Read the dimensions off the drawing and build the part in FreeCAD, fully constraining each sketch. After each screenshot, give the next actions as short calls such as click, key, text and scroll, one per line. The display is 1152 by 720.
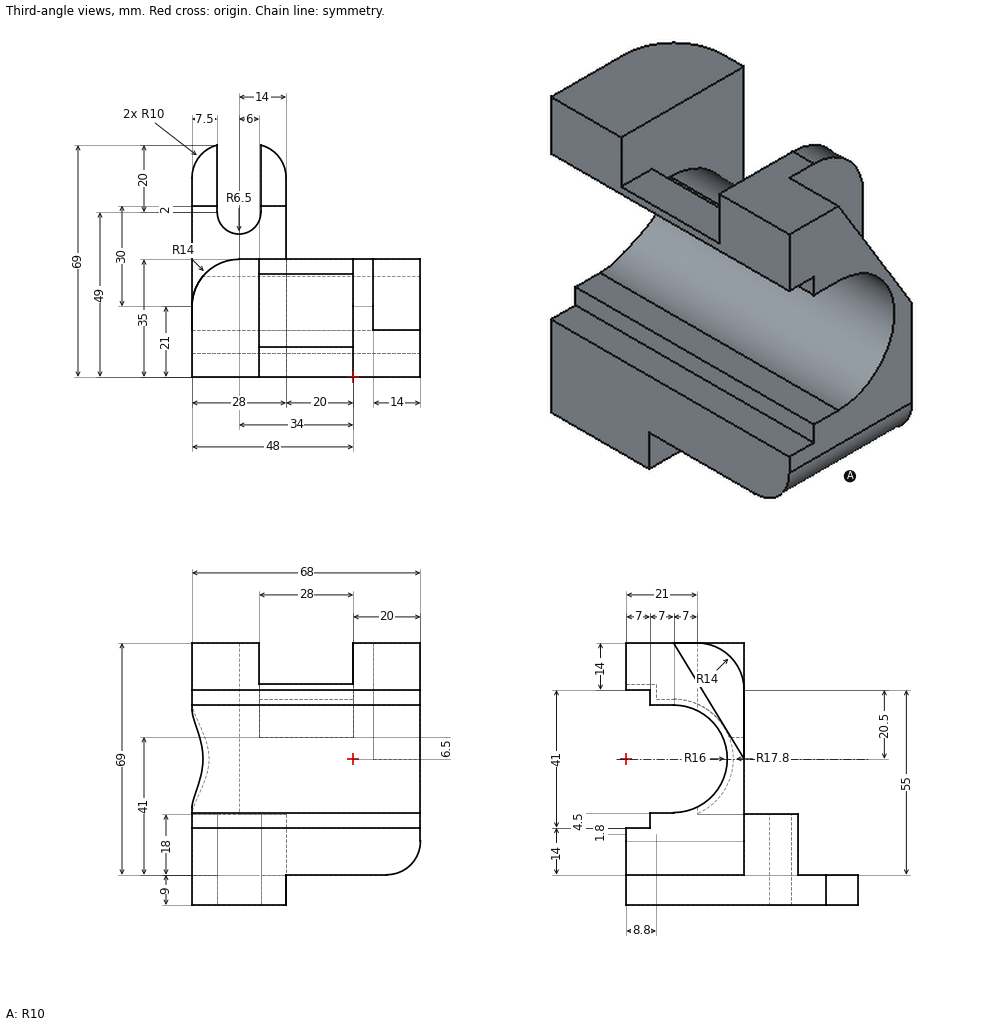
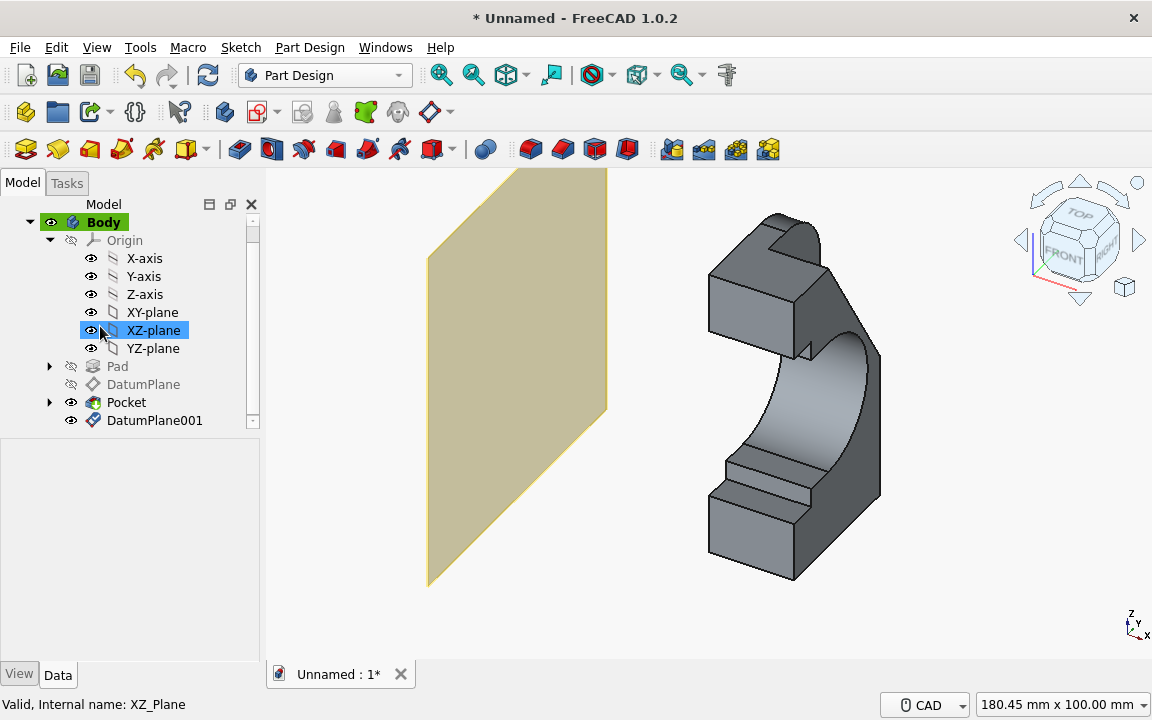
click(116, 420)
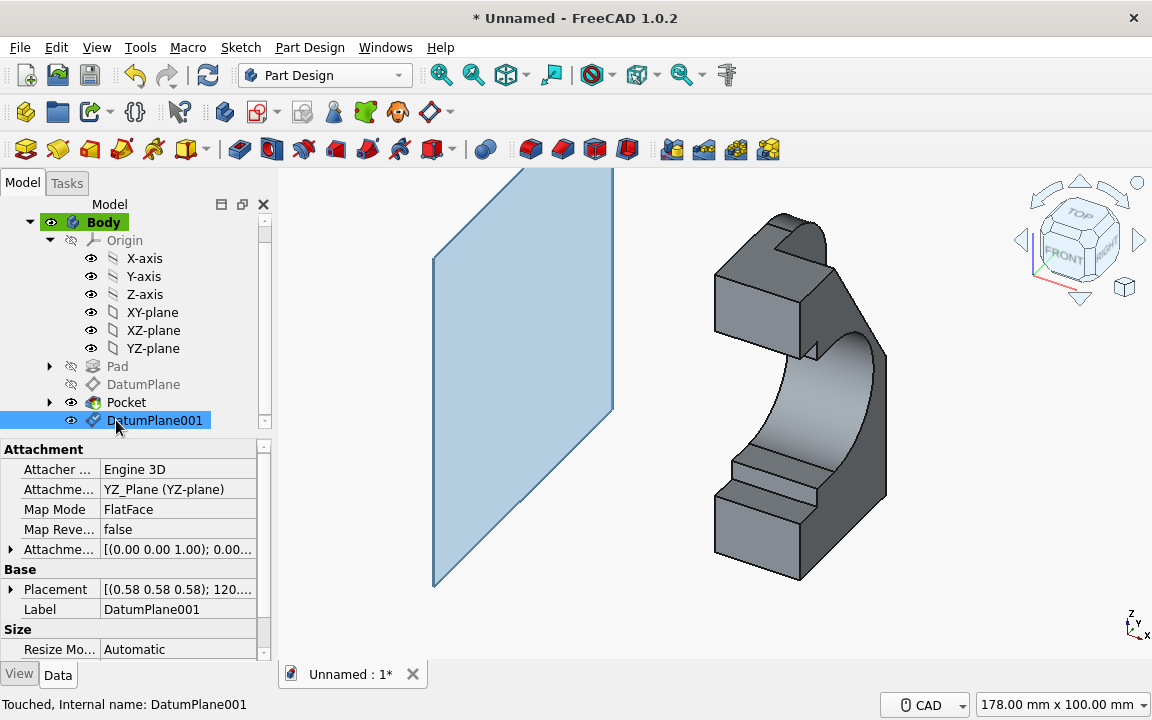
click(258, 112)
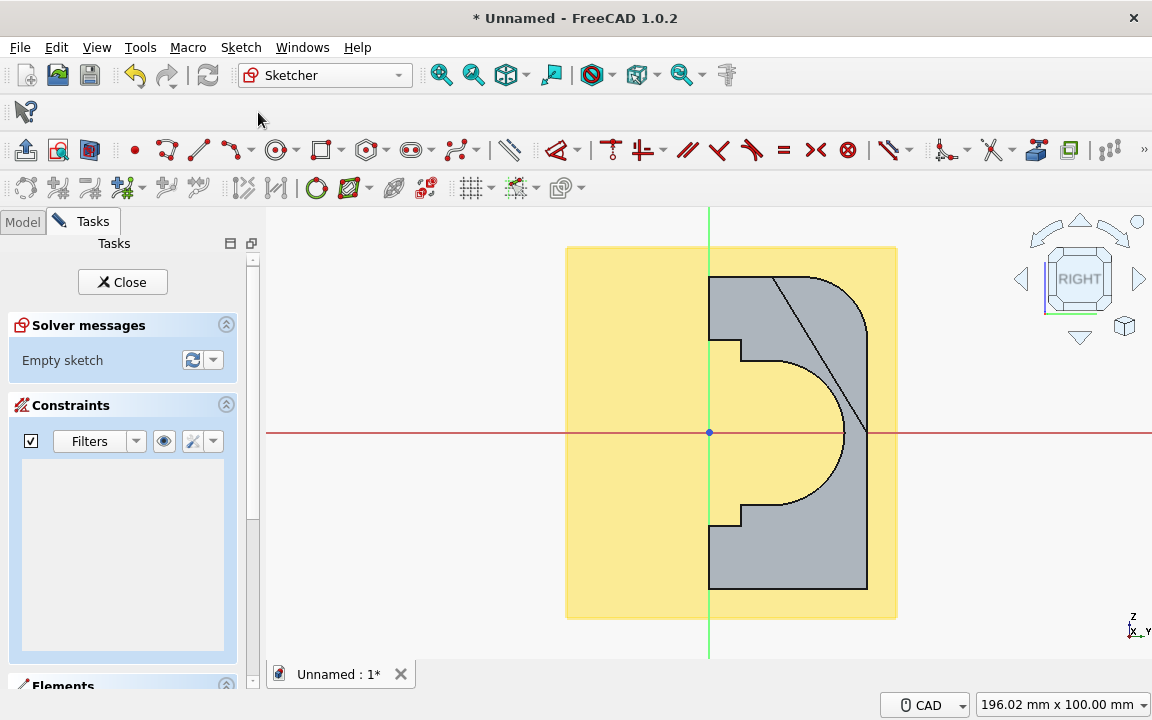
key(q)
key(s)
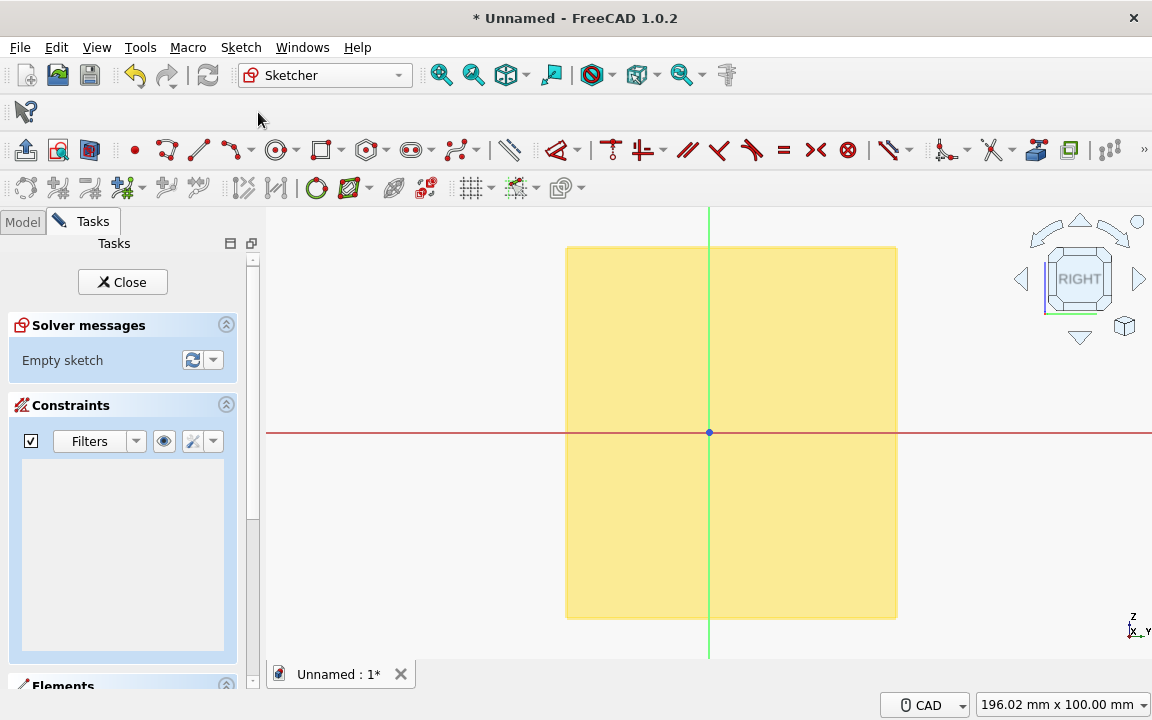
scroll(987, 433, up, 2)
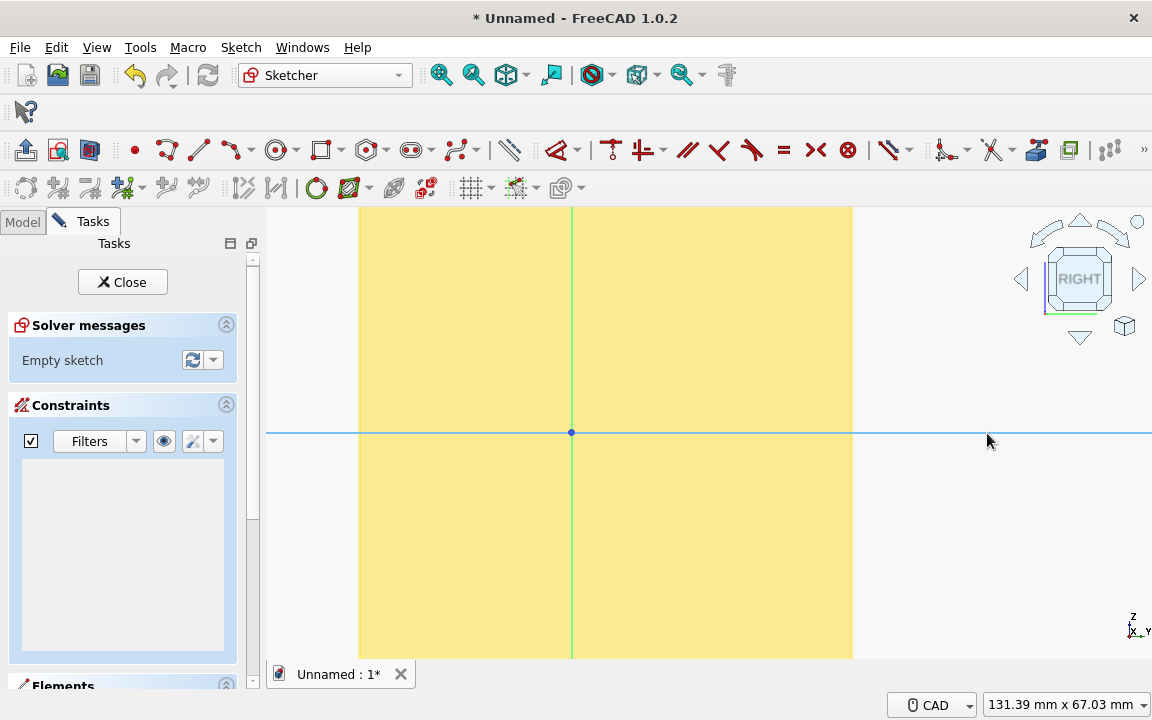
key(g)
key(m)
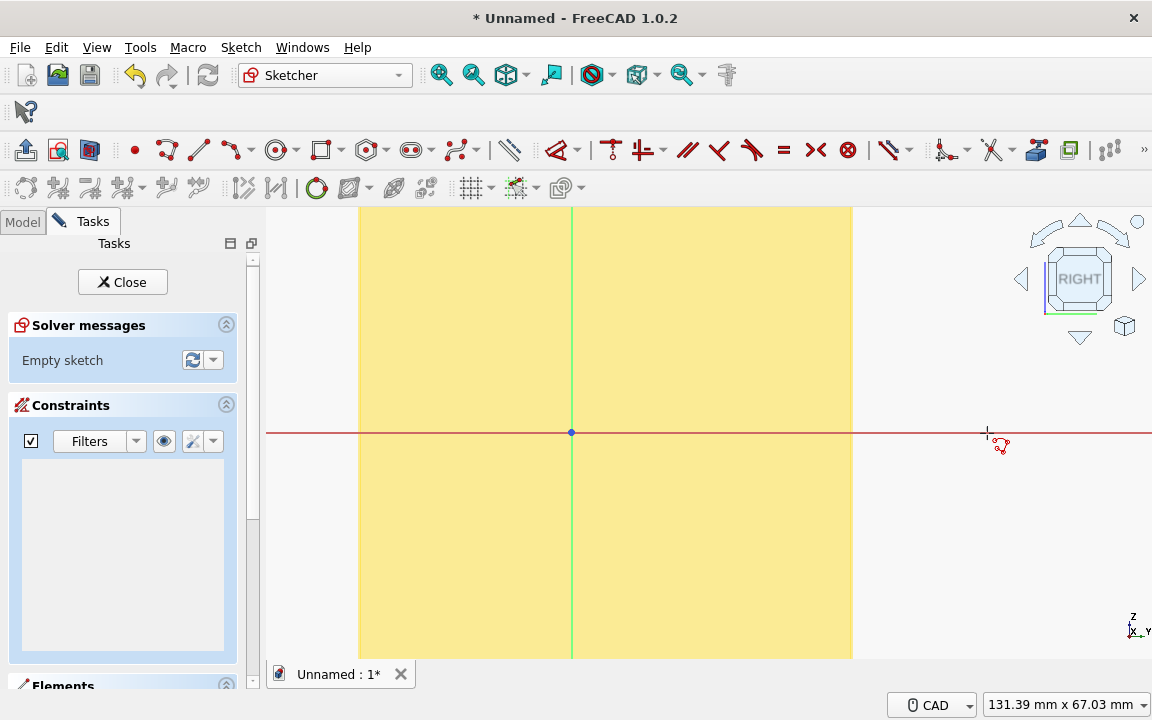
click(666, 541)
click(619, 541)
click(619, 571)
click(572, 571)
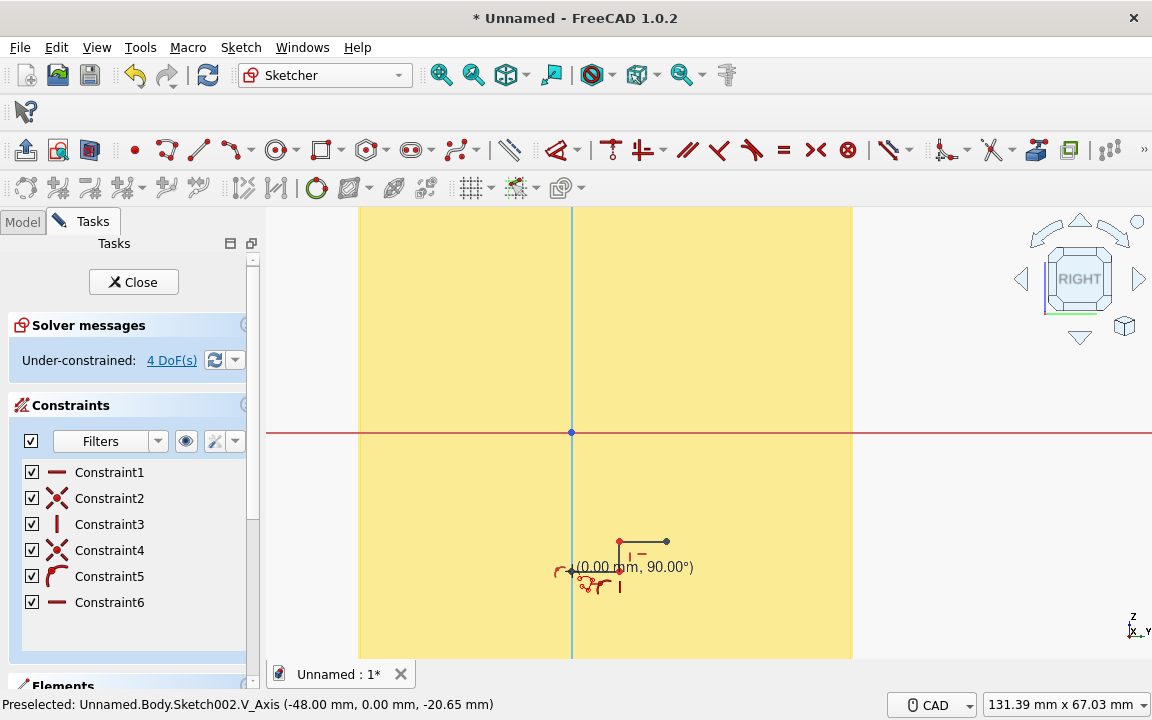
scroll(572, 583, up, 2)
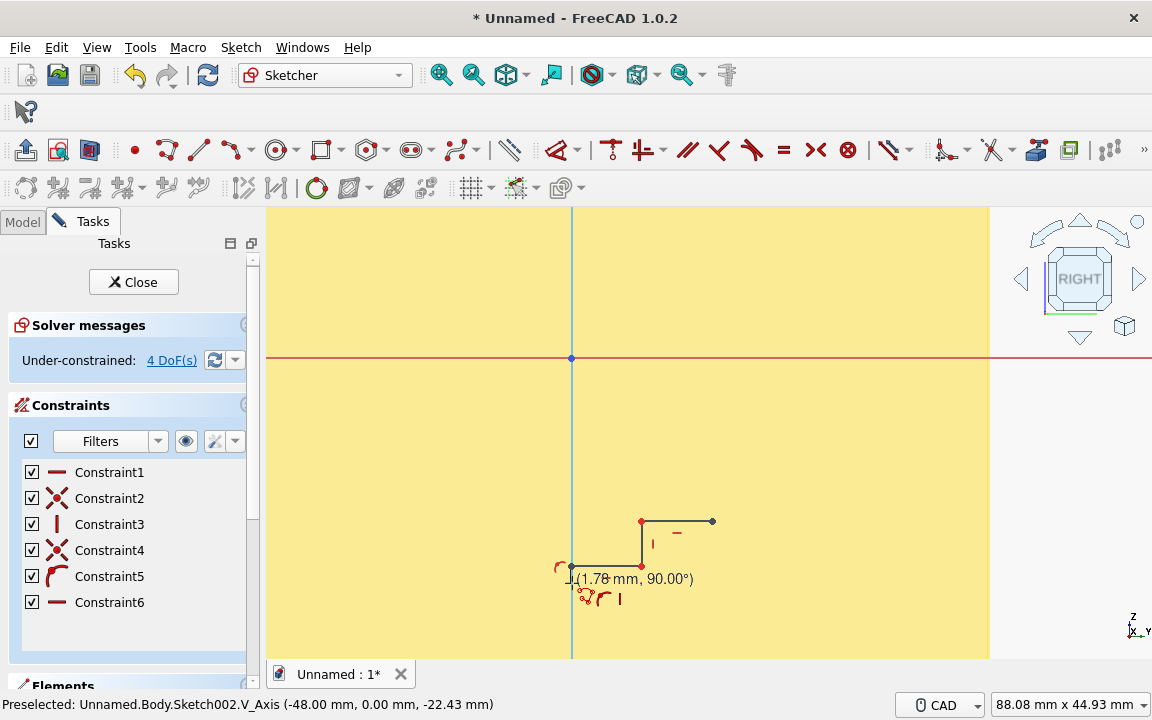
click(581, 583)
click(660, 583)
click(660, 538)
click(712, 538)
right_click(712, 538)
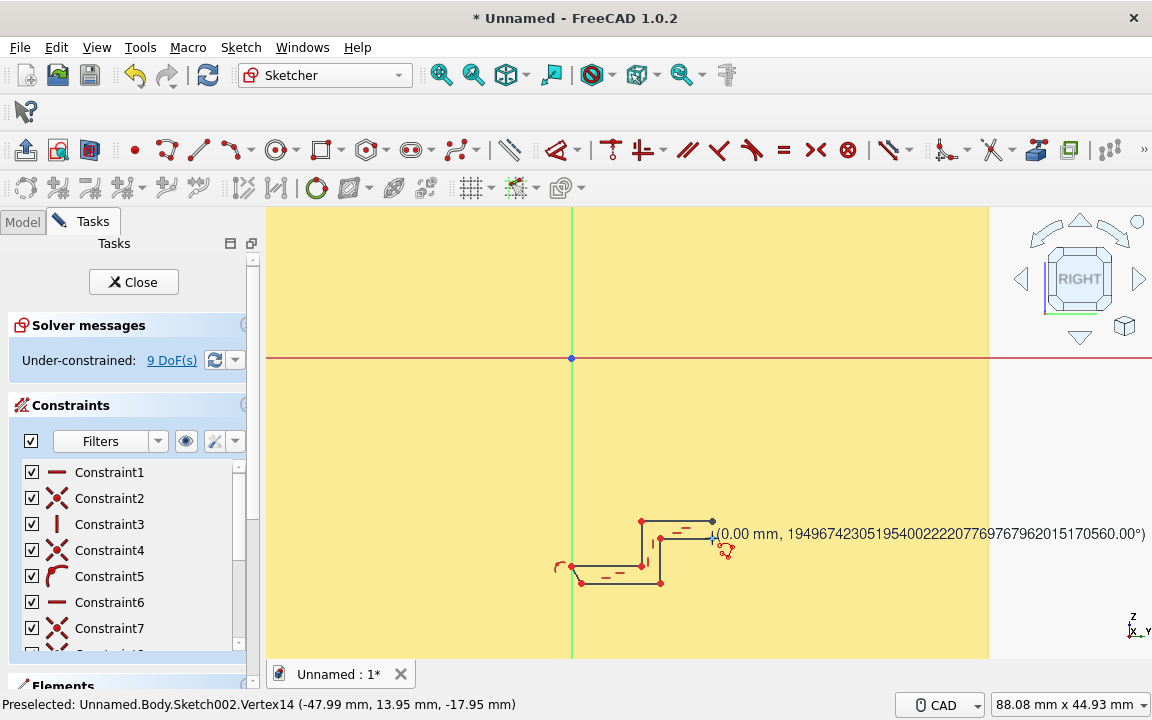
scroll(455, 585, down, 2)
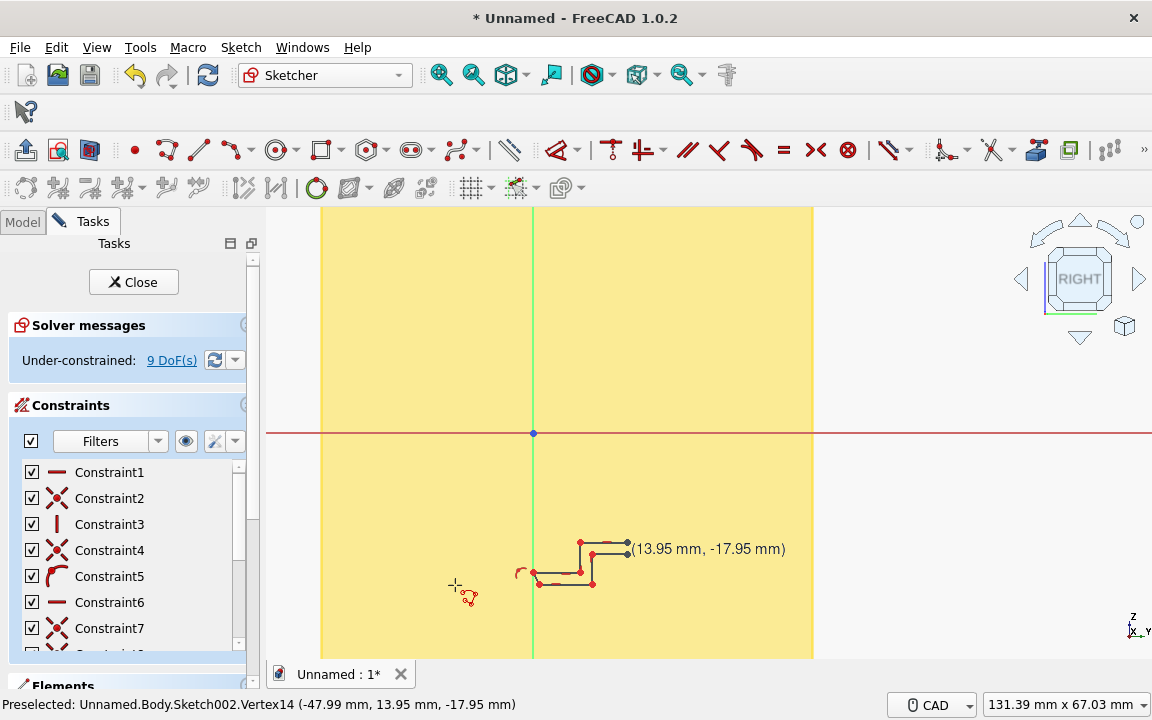
click(628, 313)
click(593, 313)
click(593, 283)
click(533, 283)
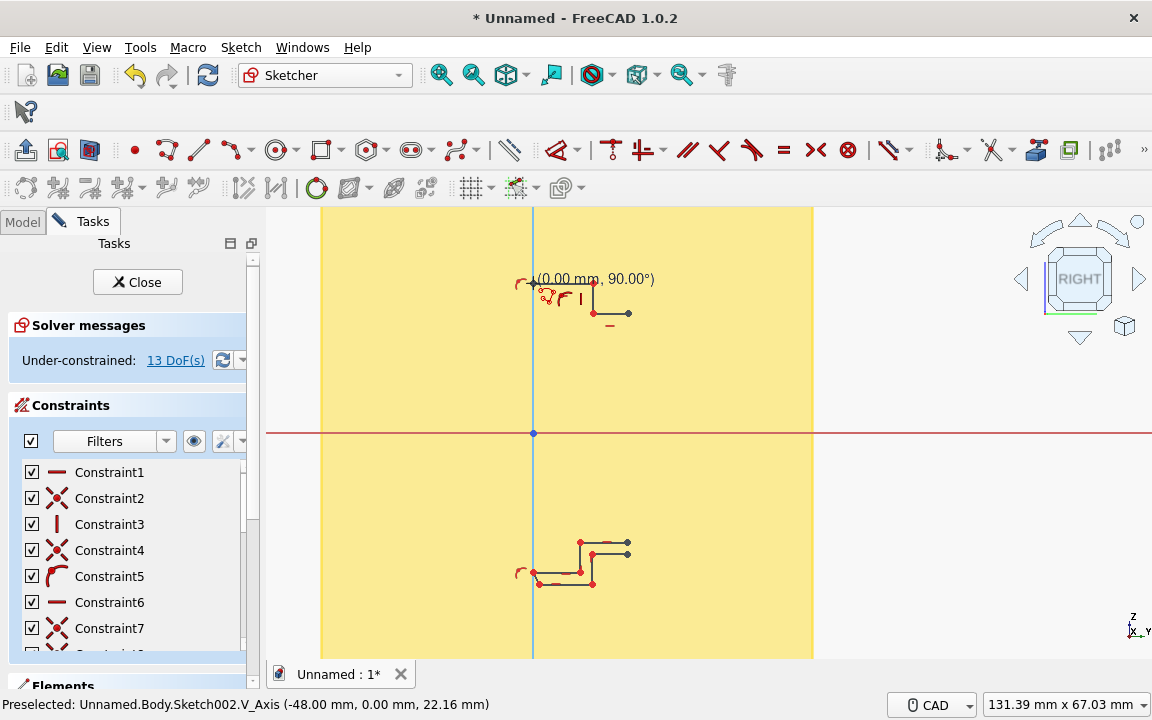
scroll(533, 295, up, 2)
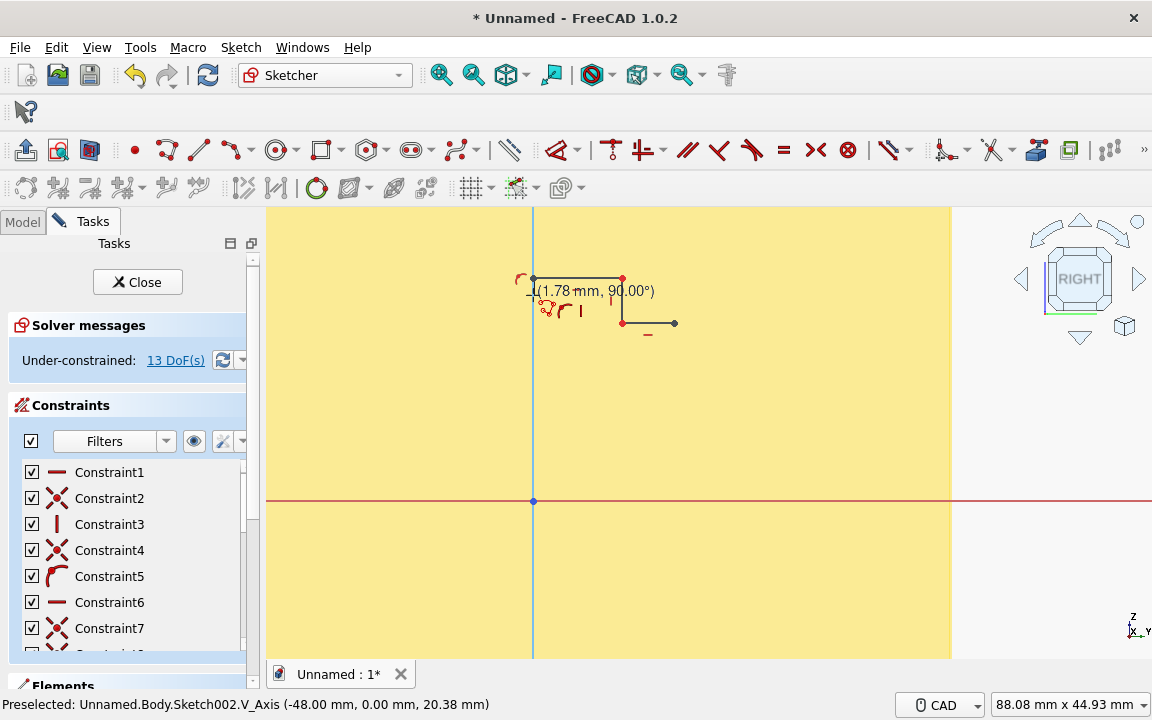
click(542, 295)
click(604, 295)
click(604, 340)
click(674, 340)
right_click(674, 340)